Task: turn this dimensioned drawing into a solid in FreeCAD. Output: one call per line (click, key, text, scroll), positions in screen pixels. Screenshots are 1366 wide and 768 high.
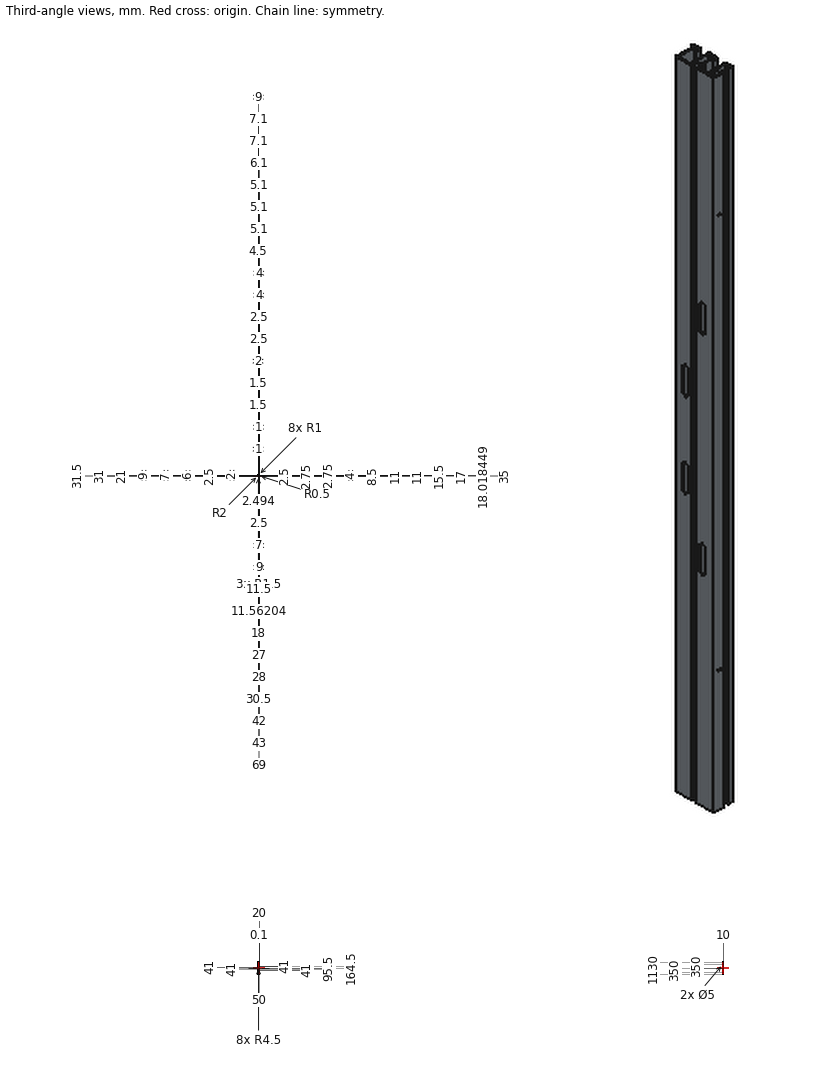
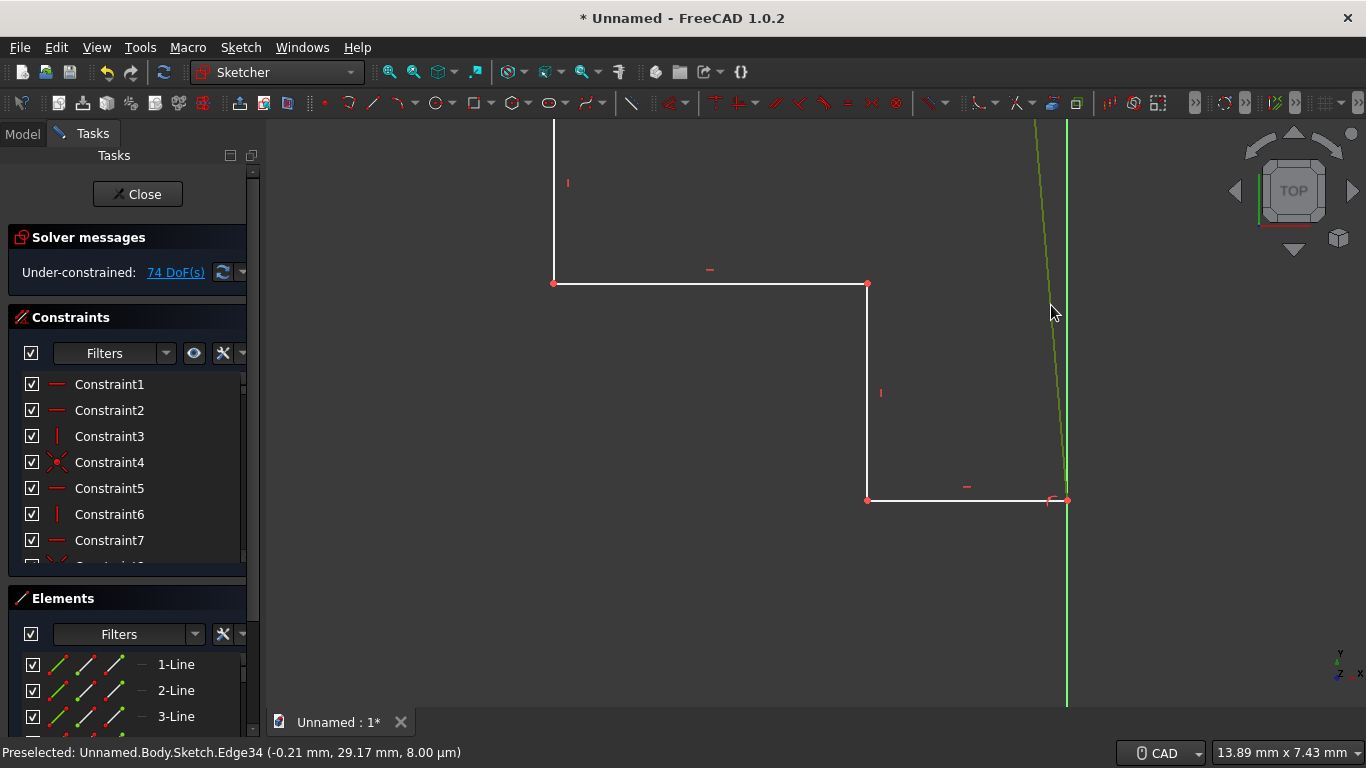
click(758, 104)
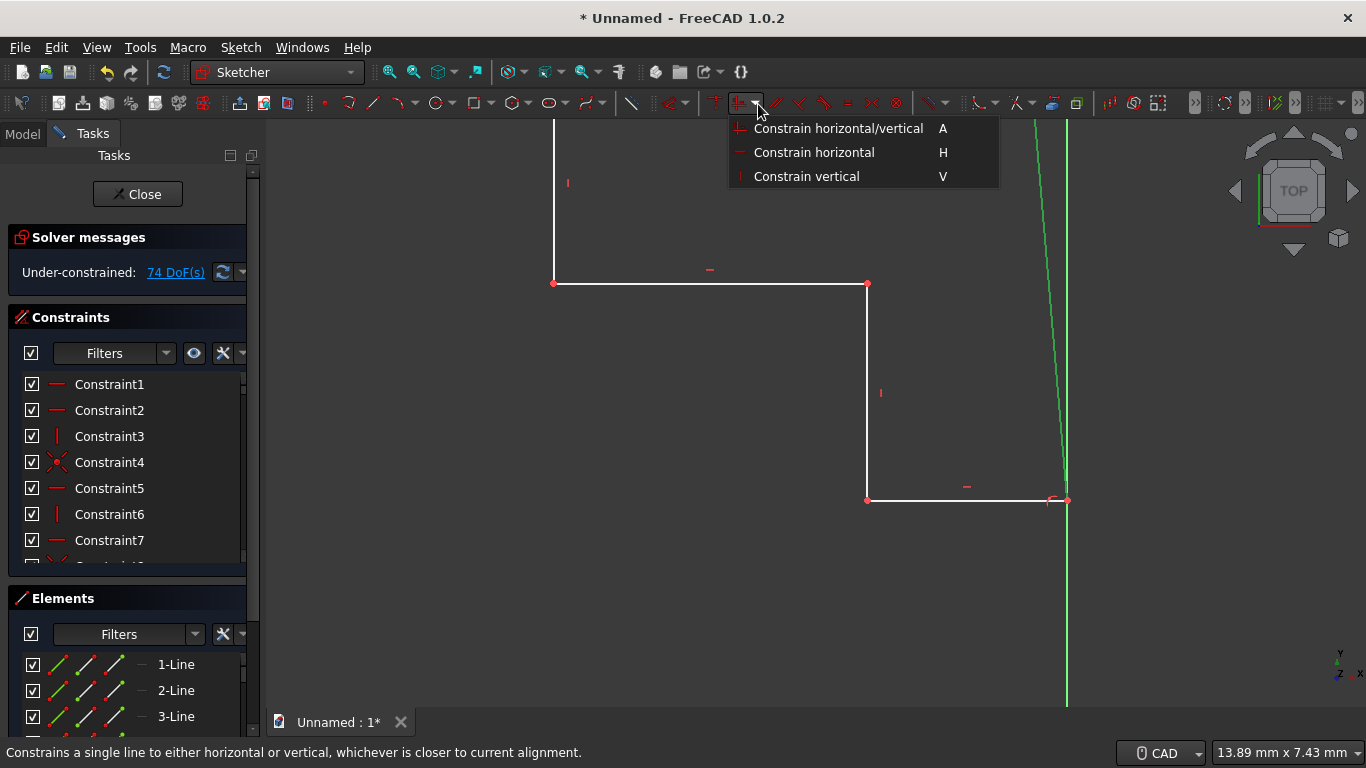
click(864, 176)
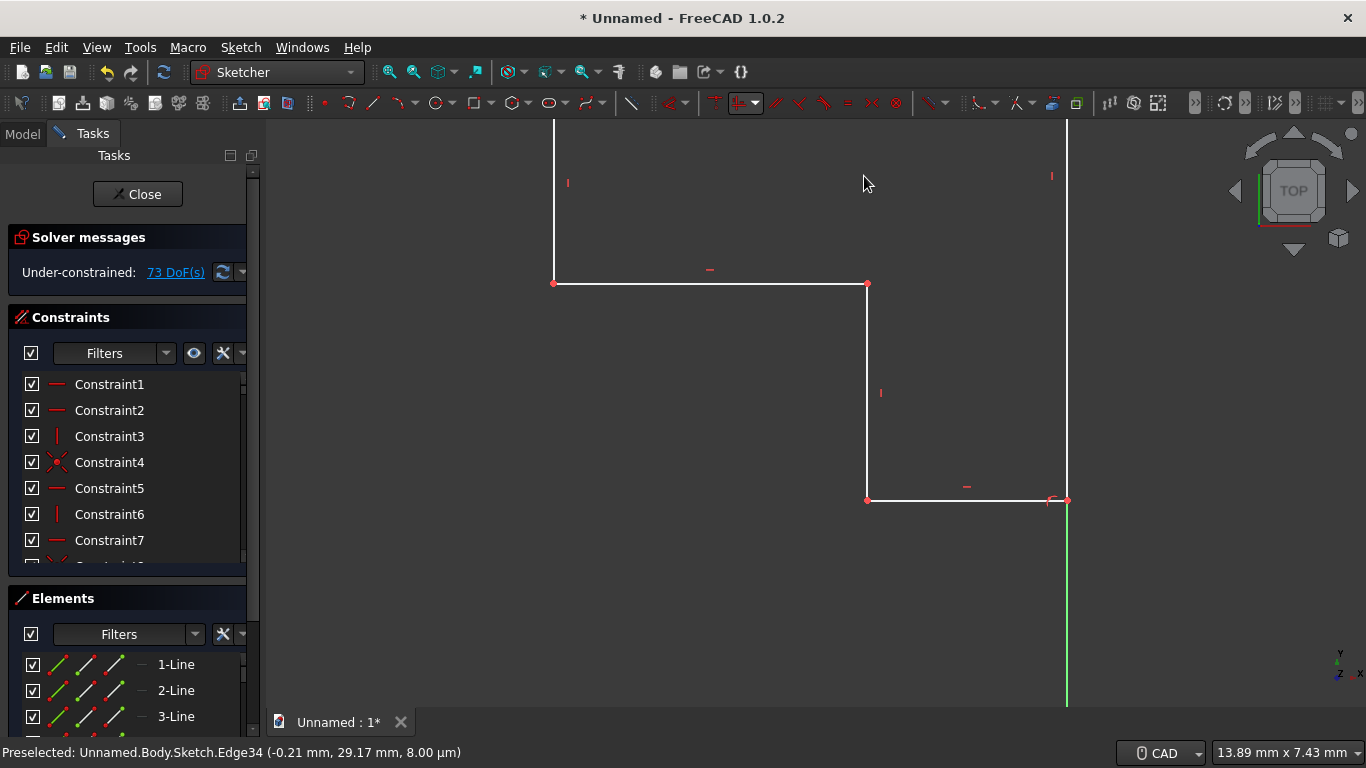
scroll(1053, 311, down, 11)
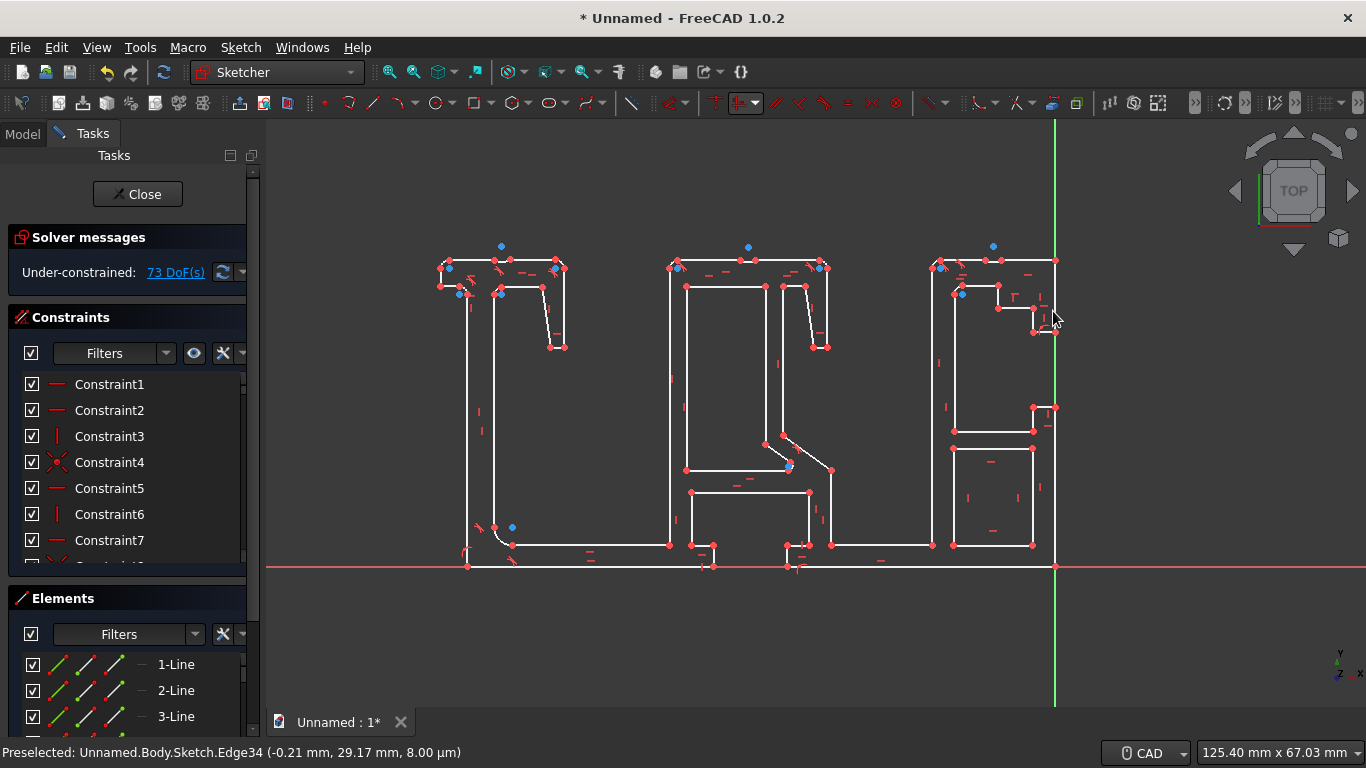
scroll(674, 261, up, 7)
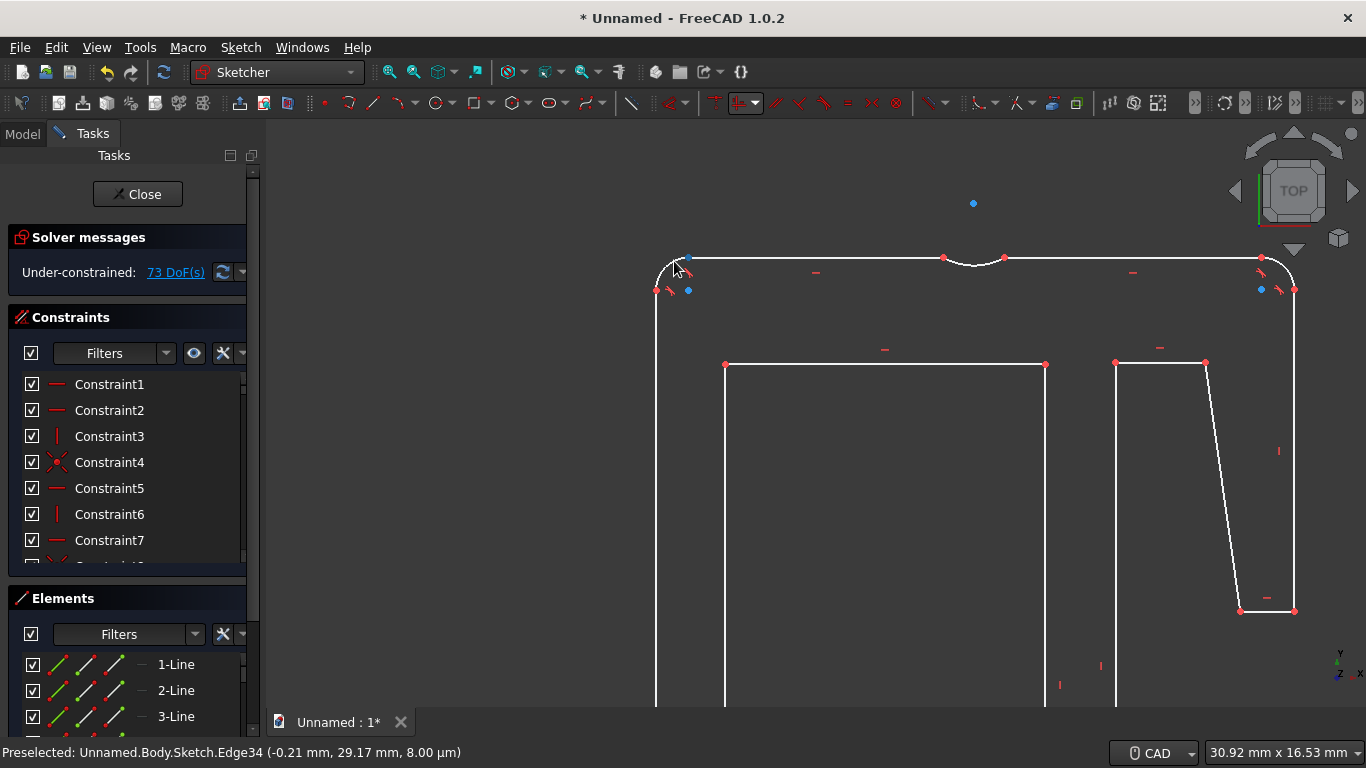
click(674, 261)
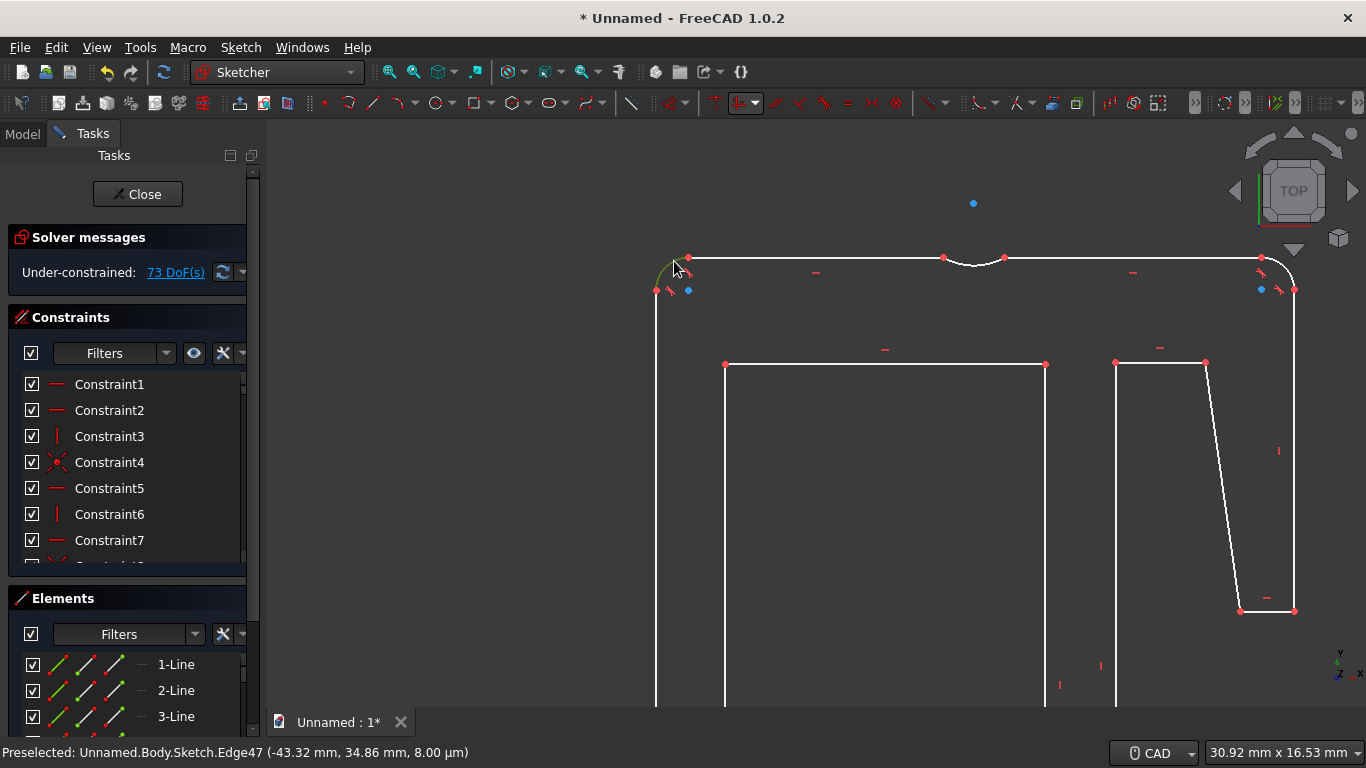
scroll(673, 261, down, 7)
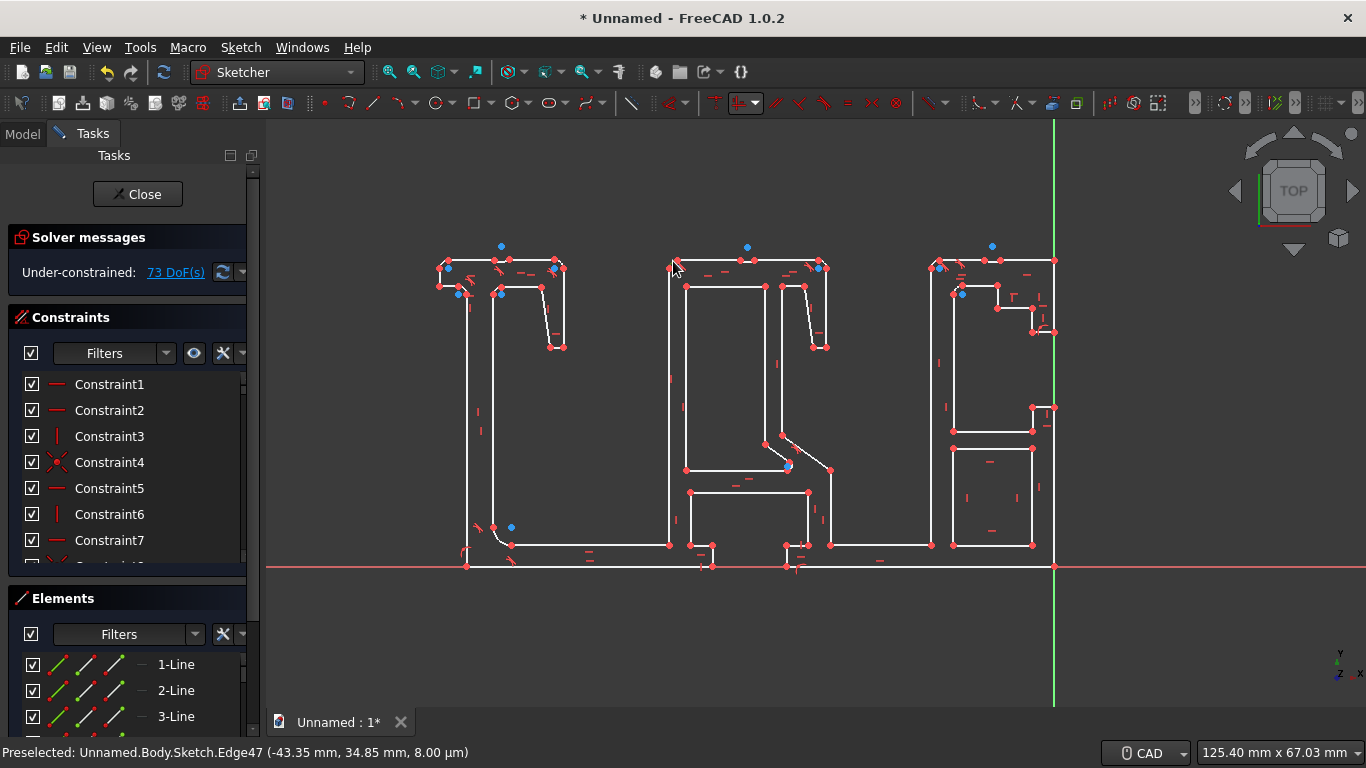
scroll(498, 288, up, 7)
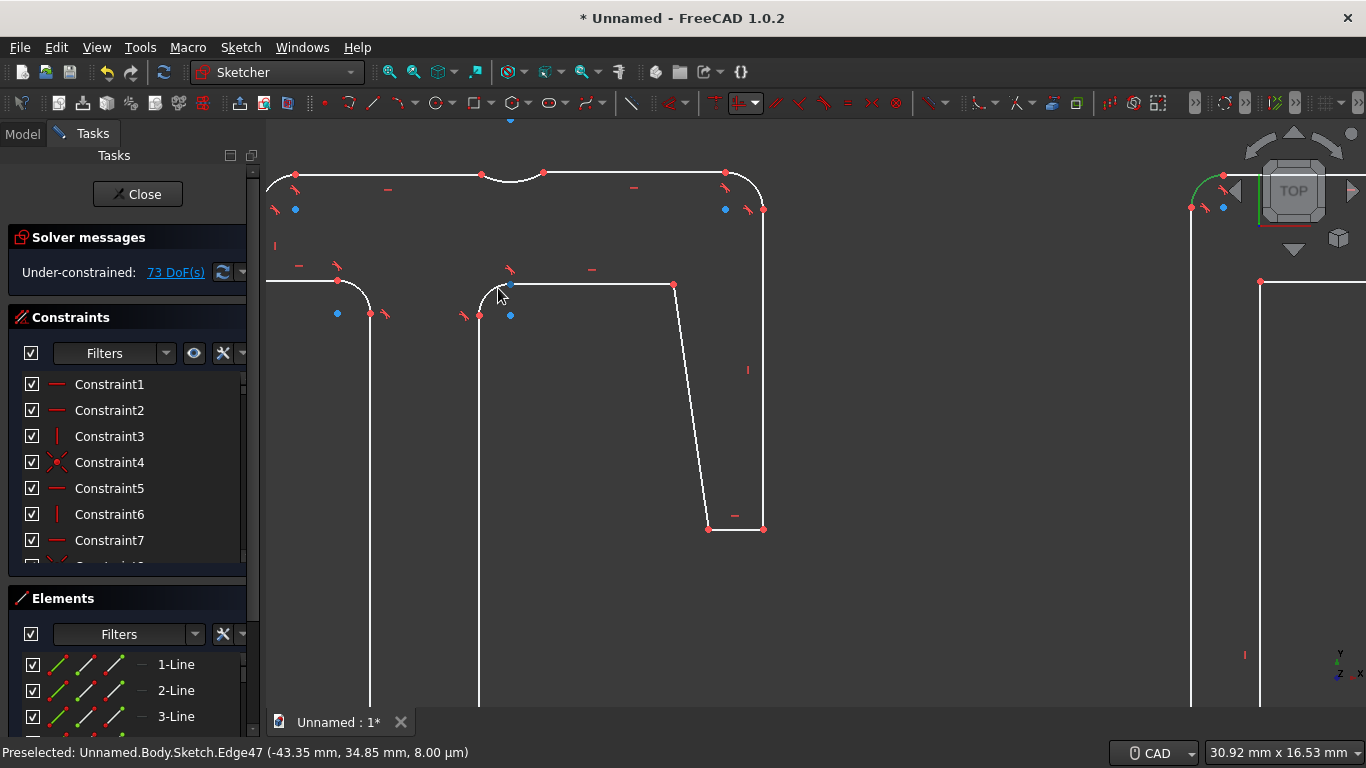
click(496, 287)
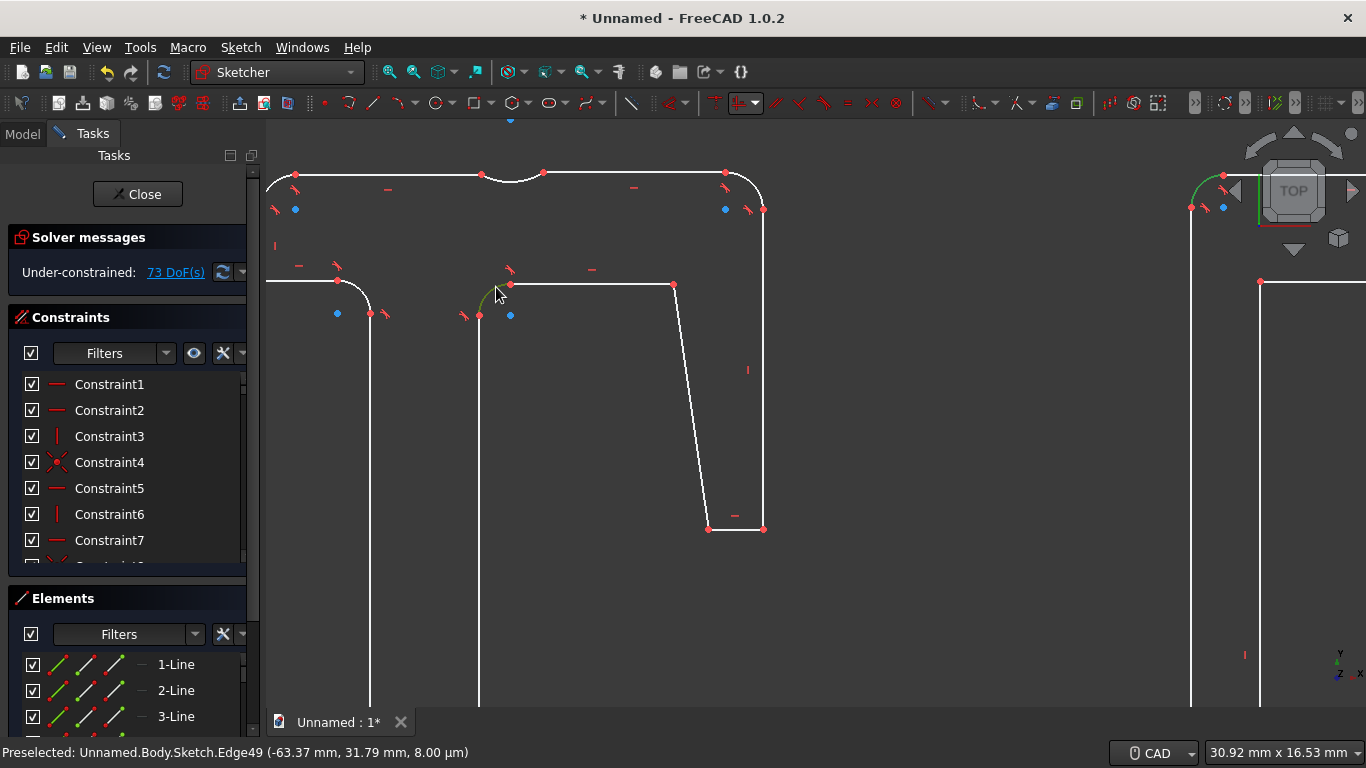
click(759, 193)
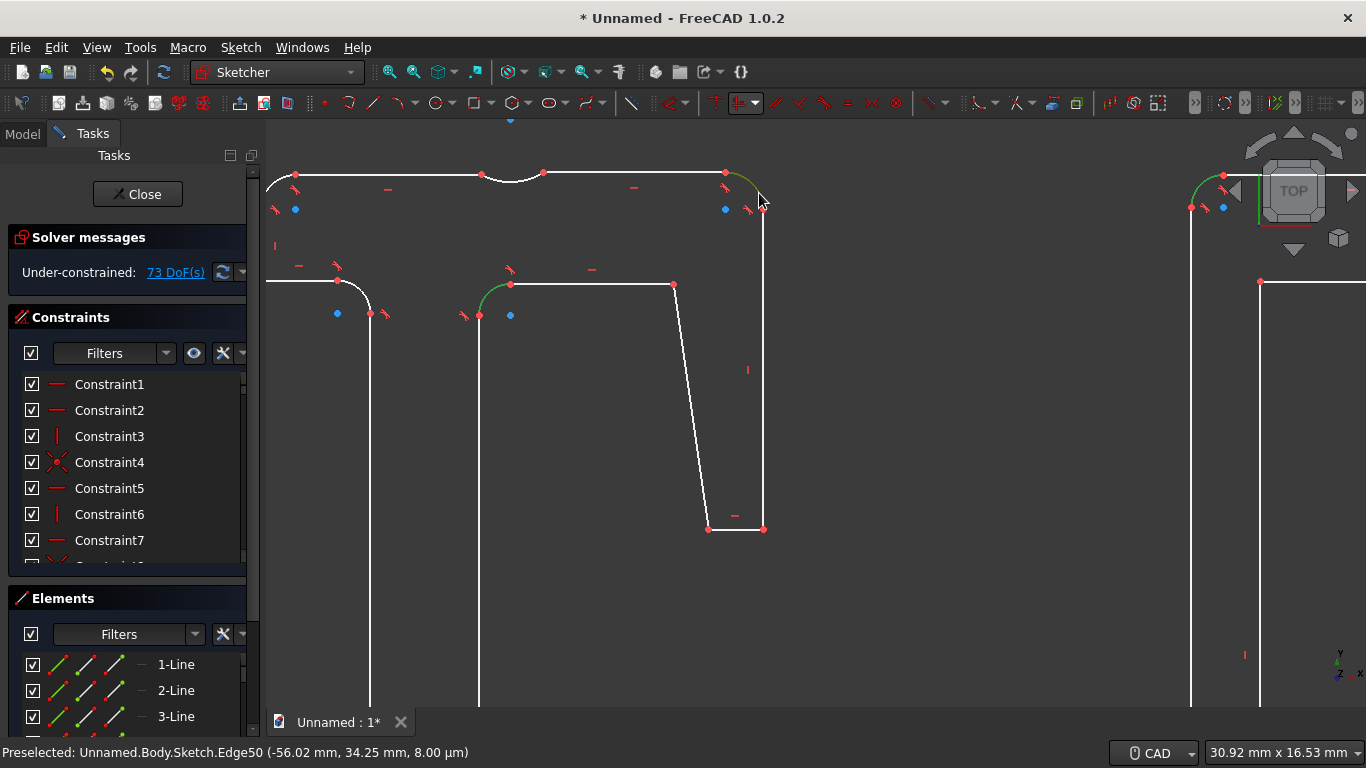
scroll(498, 288, down, 7)